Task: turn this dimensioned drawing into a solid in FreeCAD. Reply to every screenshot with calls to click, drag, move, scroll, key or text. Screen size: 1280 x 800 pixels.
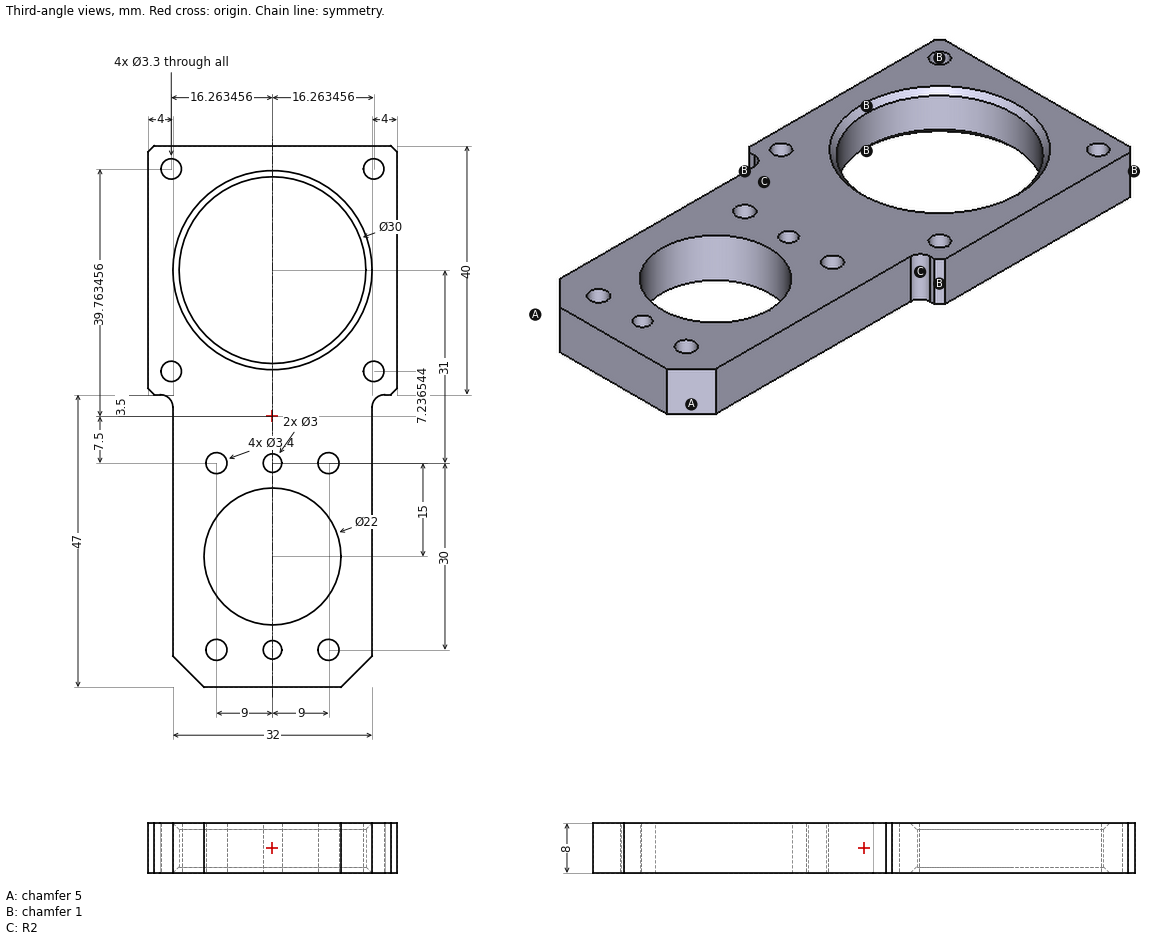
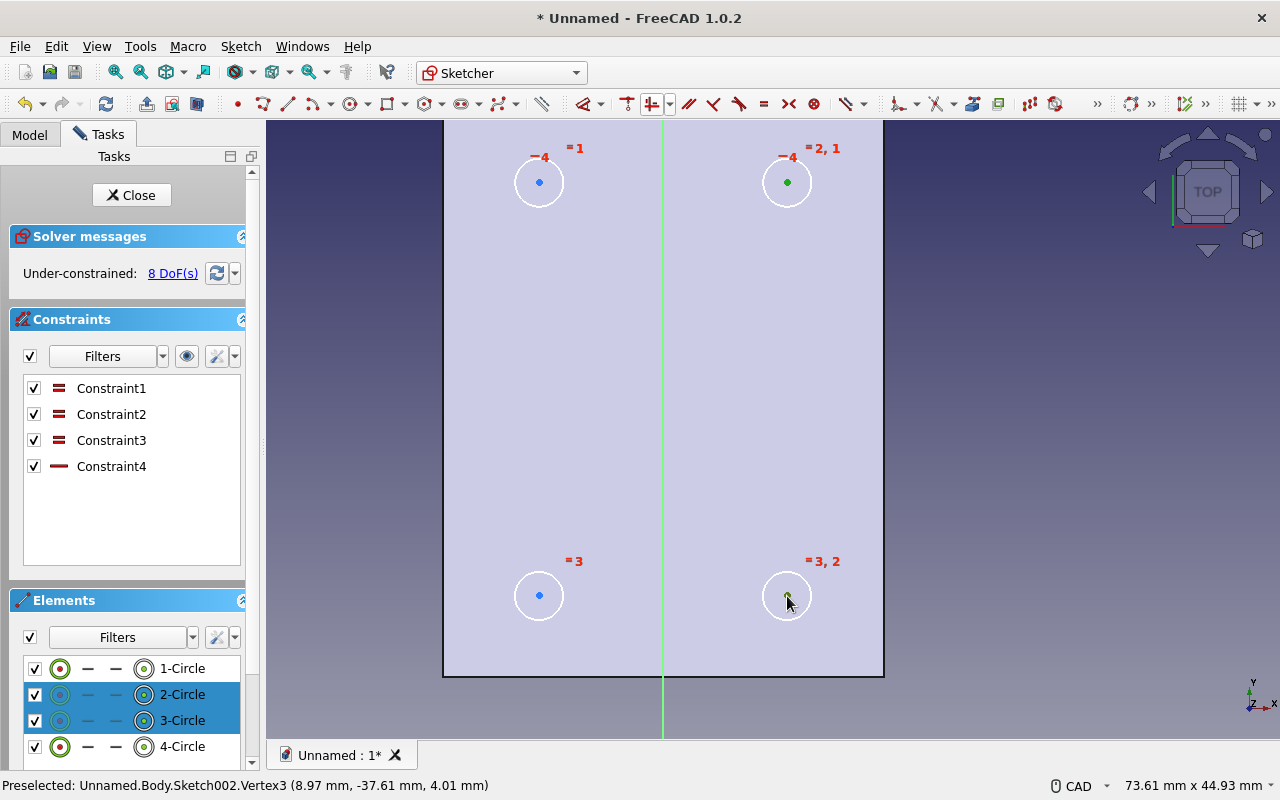
key(v)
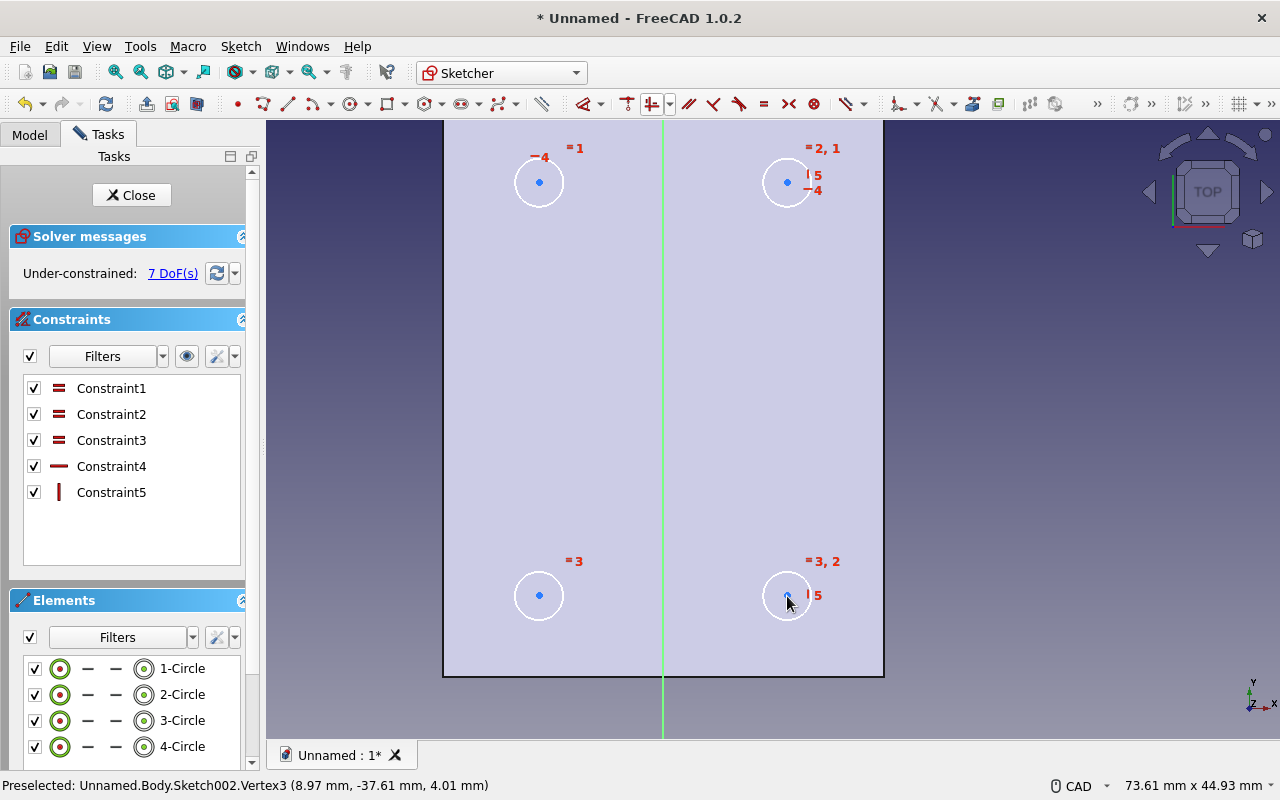
click(539, 183)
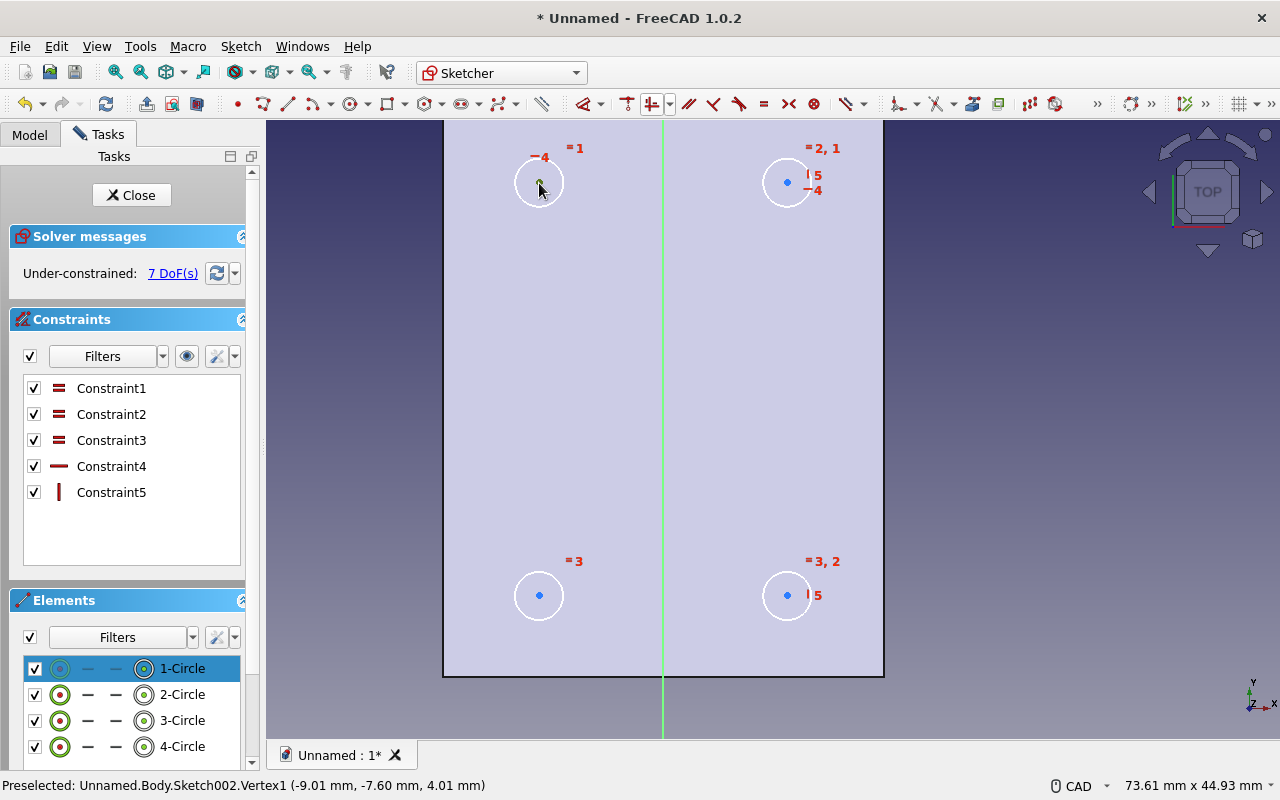
click(539, 596)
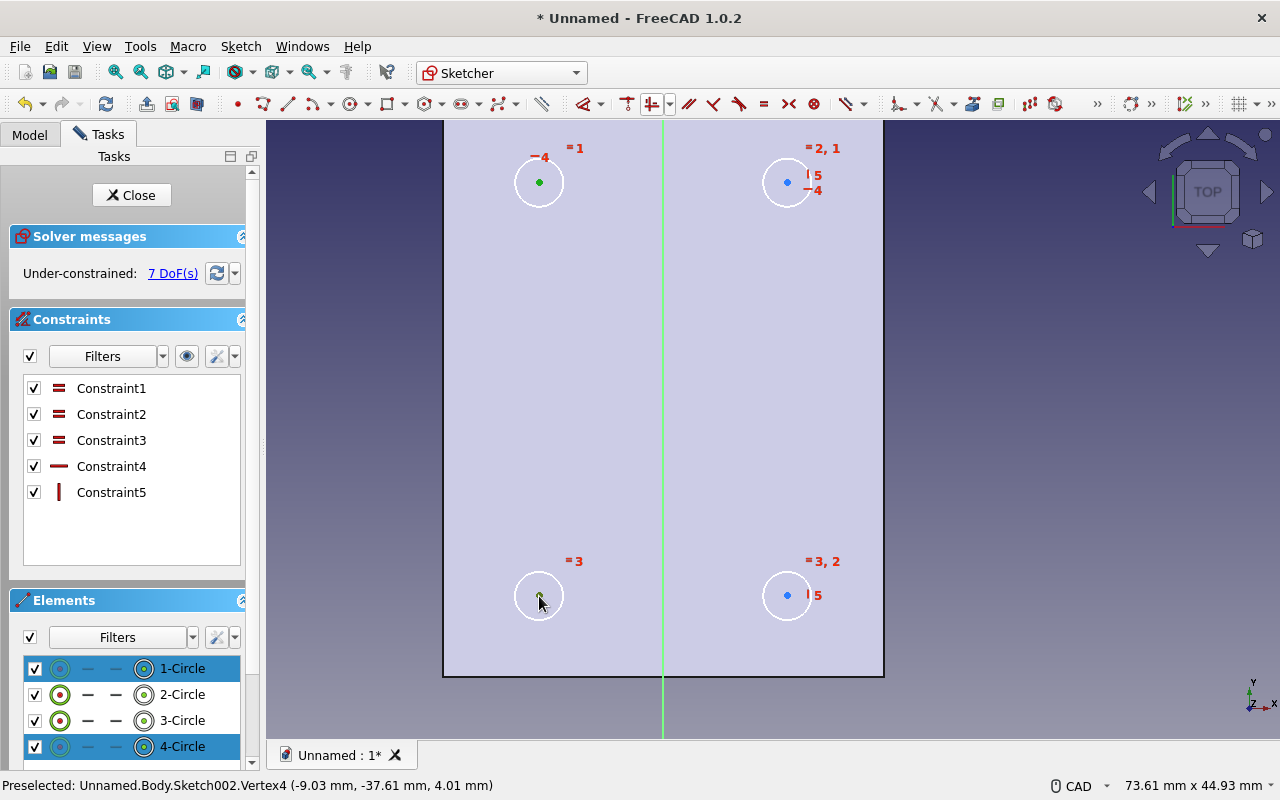
key(v)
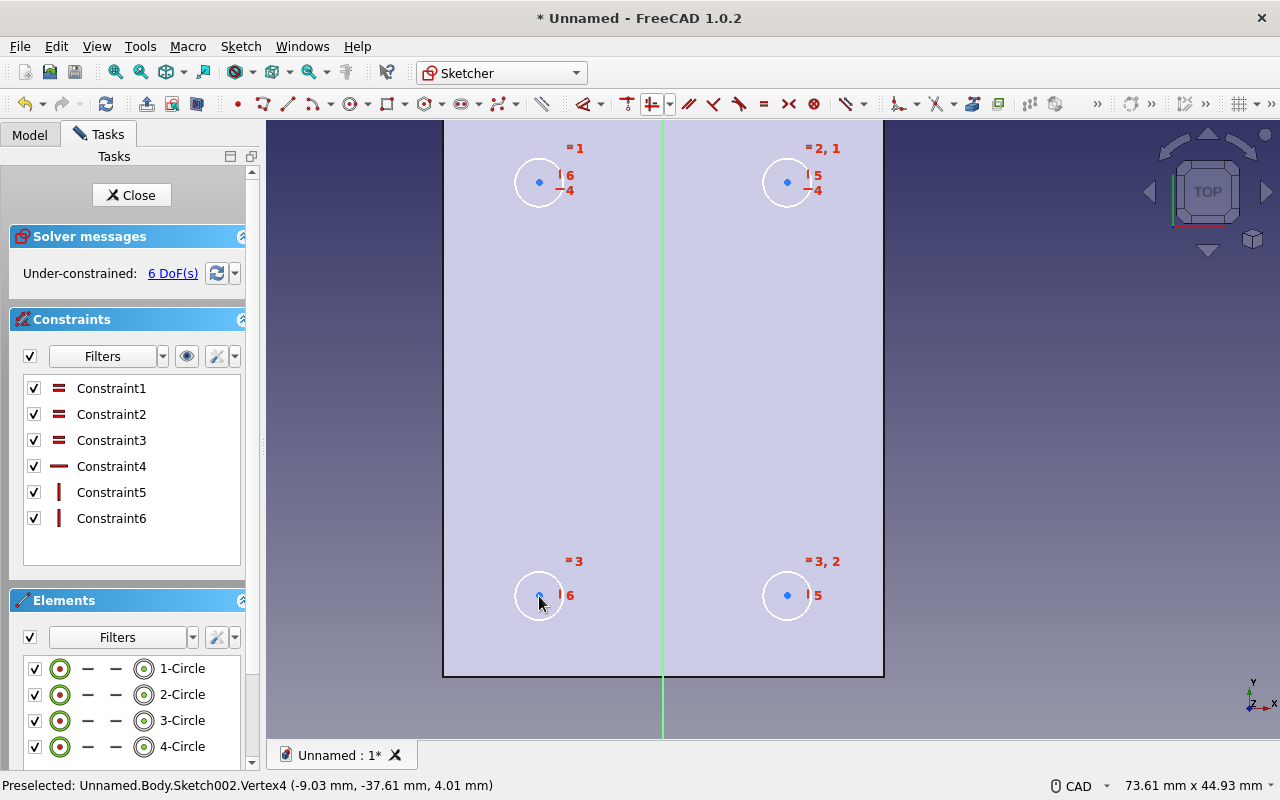
click(787, 596)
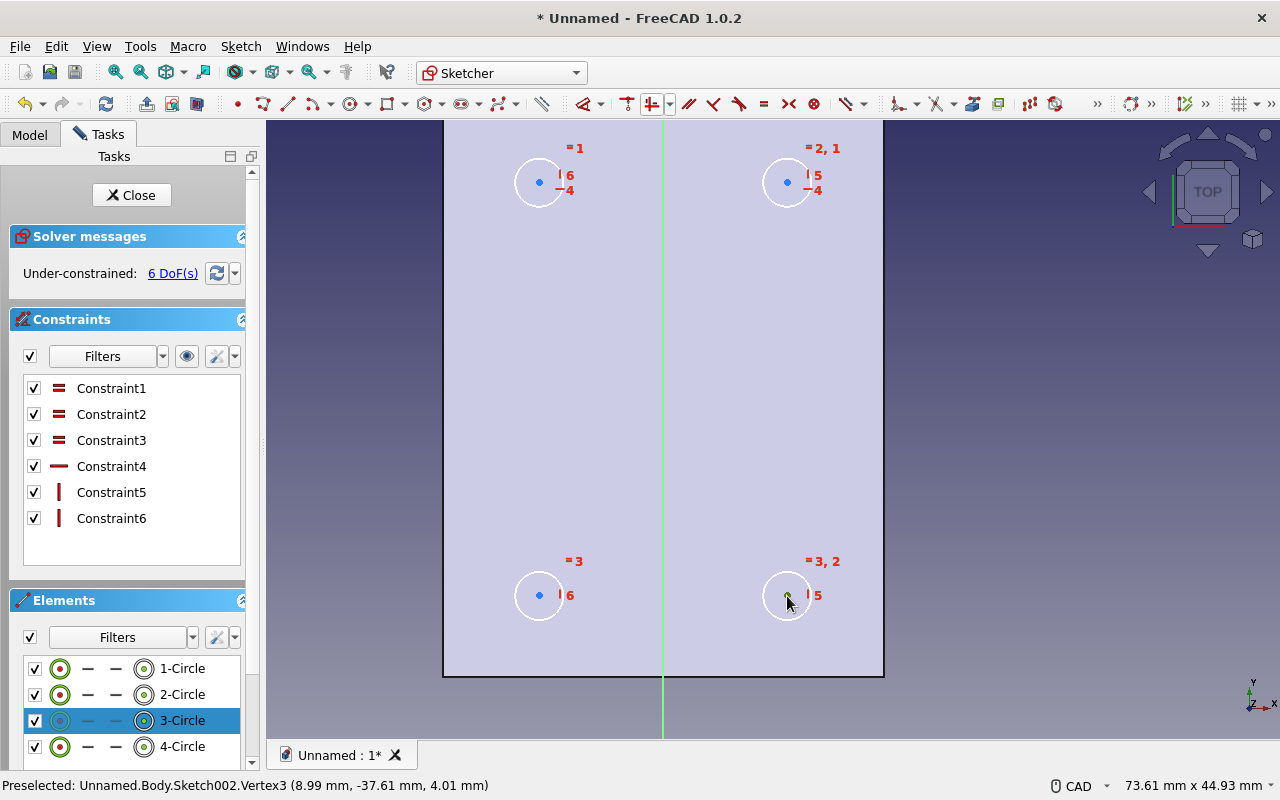
click(539, 596)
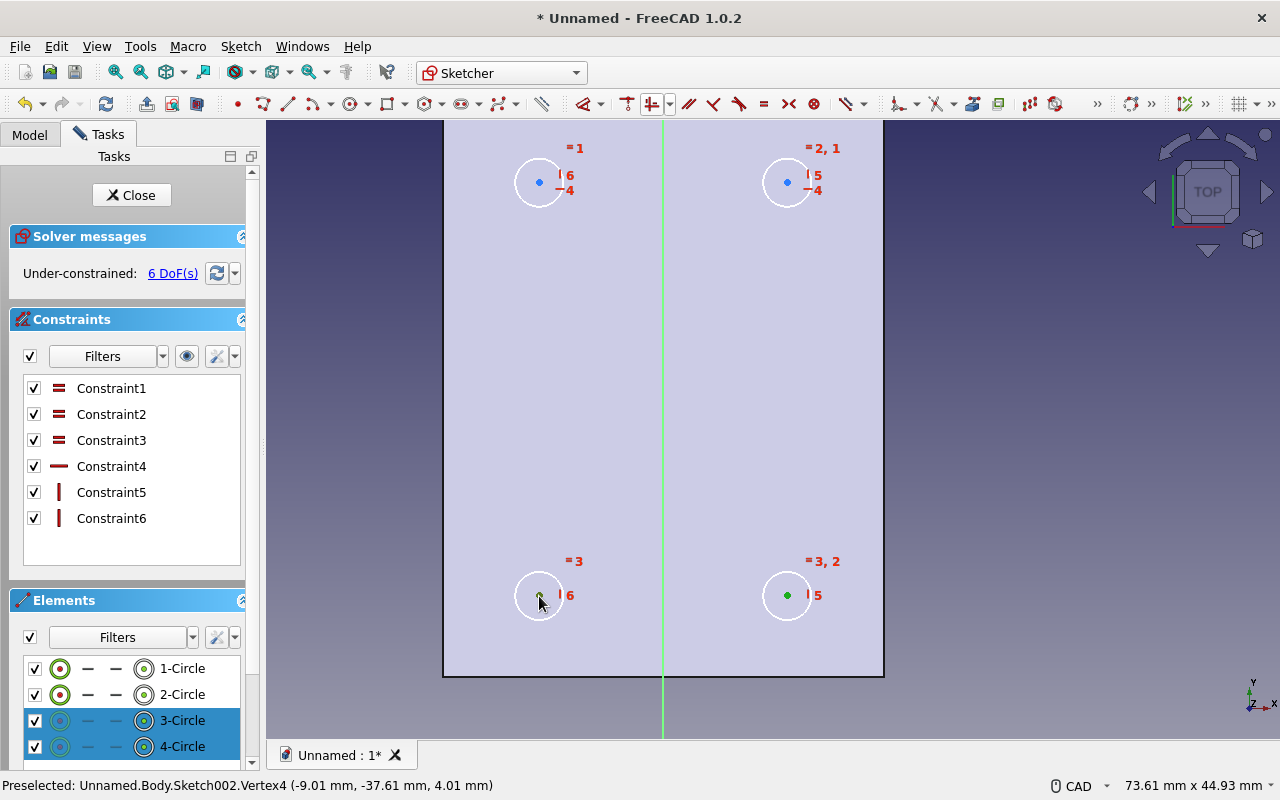
key(h)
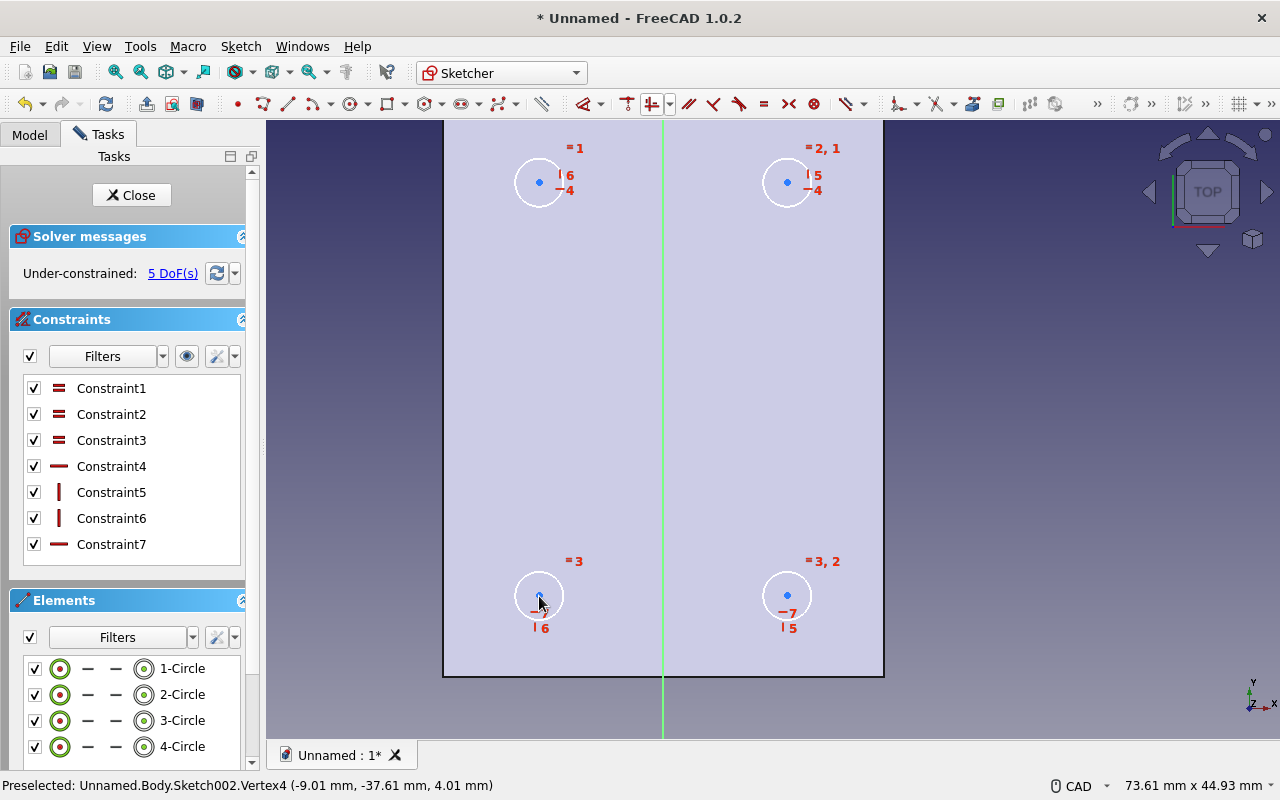
key(d)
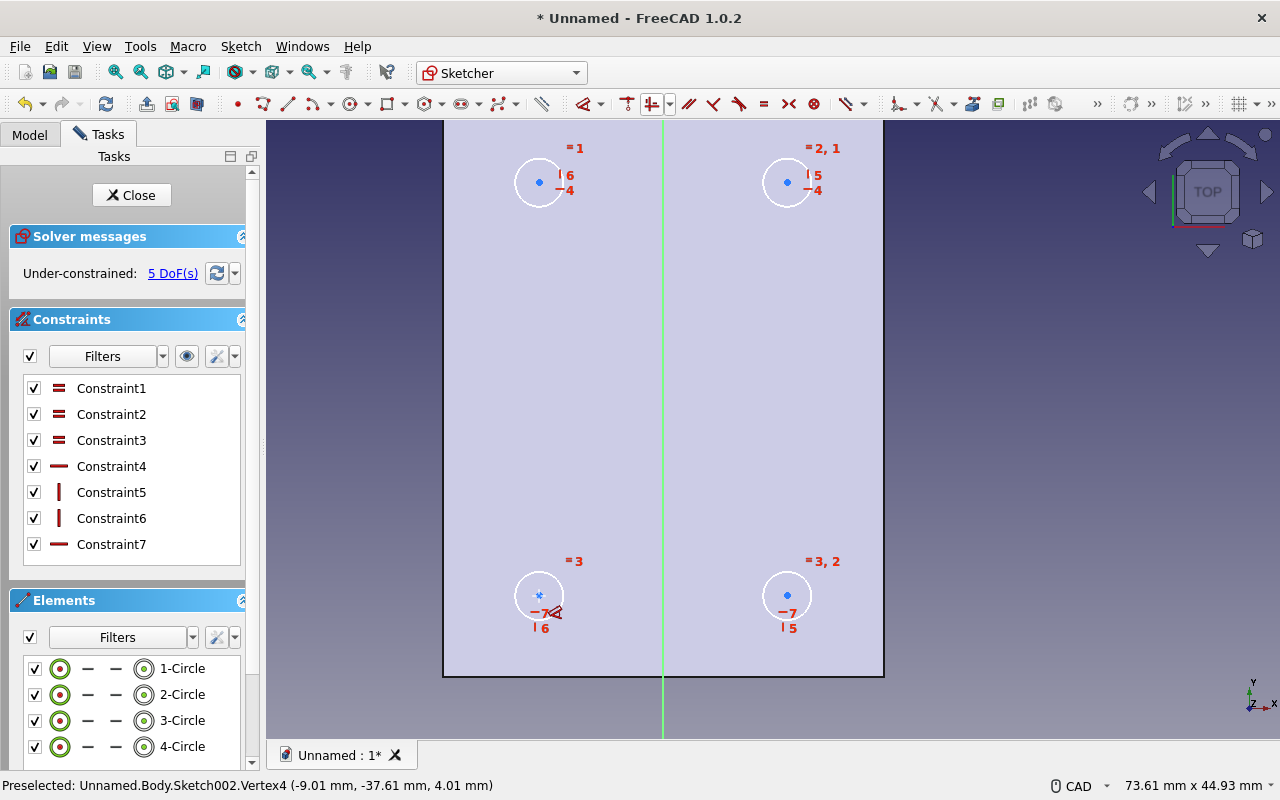
click(556, 166)
click(593, 167)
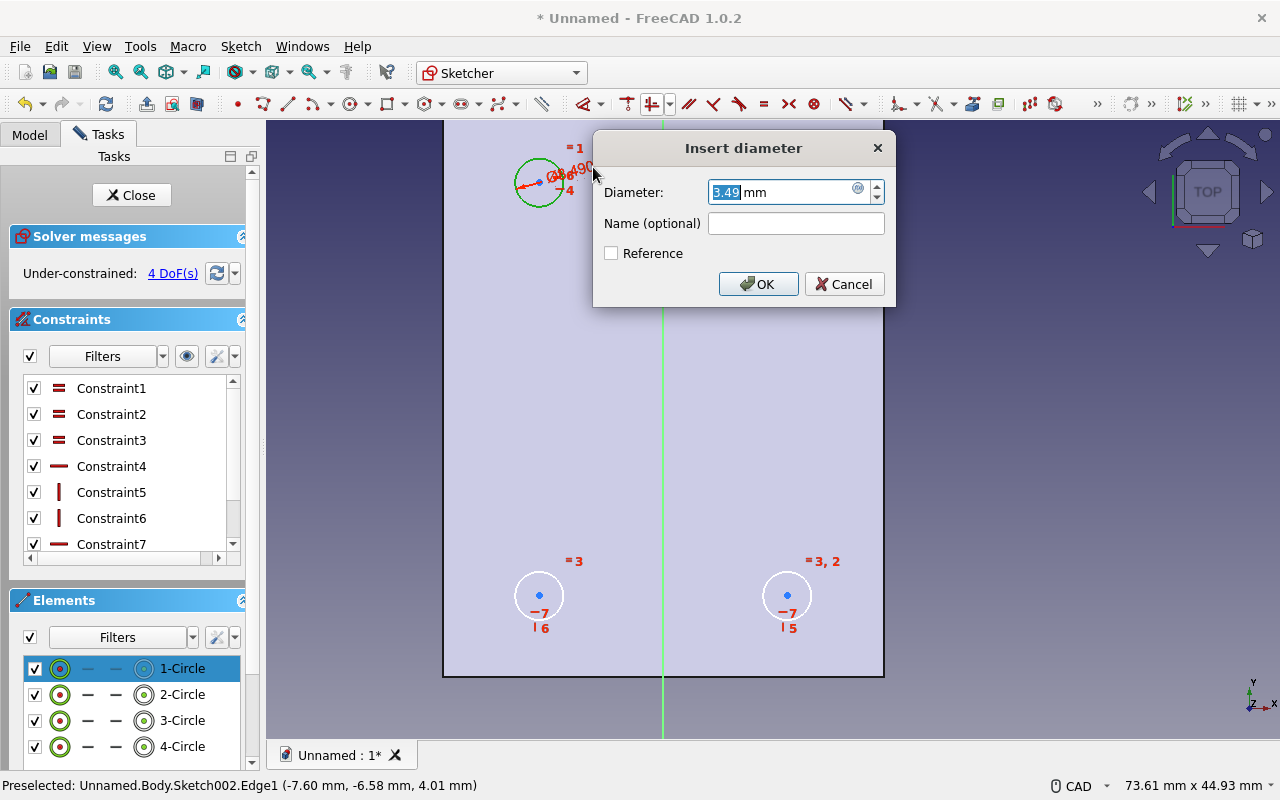
text(3.4)
key(Return)